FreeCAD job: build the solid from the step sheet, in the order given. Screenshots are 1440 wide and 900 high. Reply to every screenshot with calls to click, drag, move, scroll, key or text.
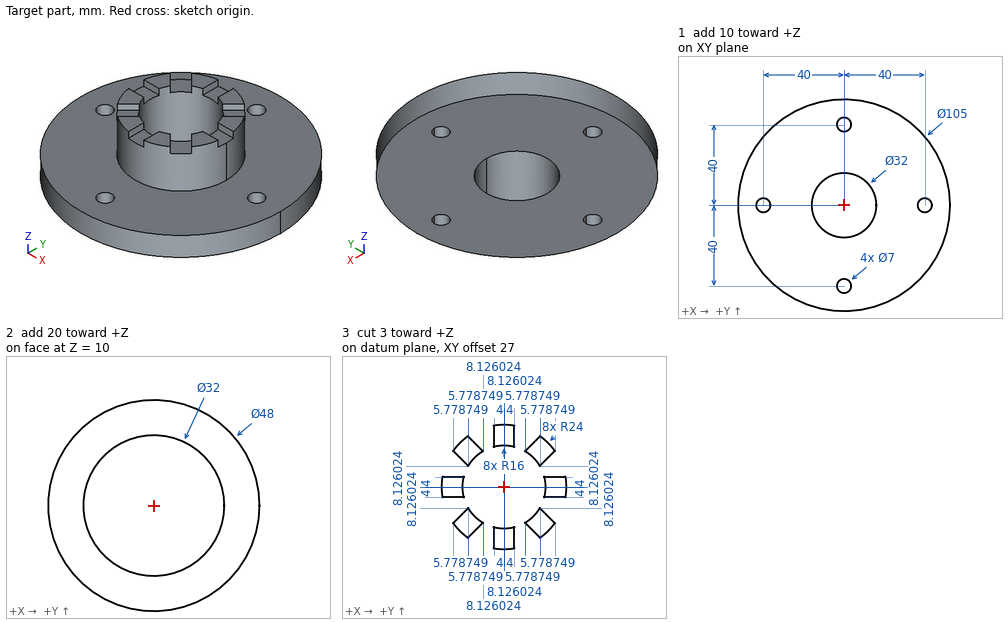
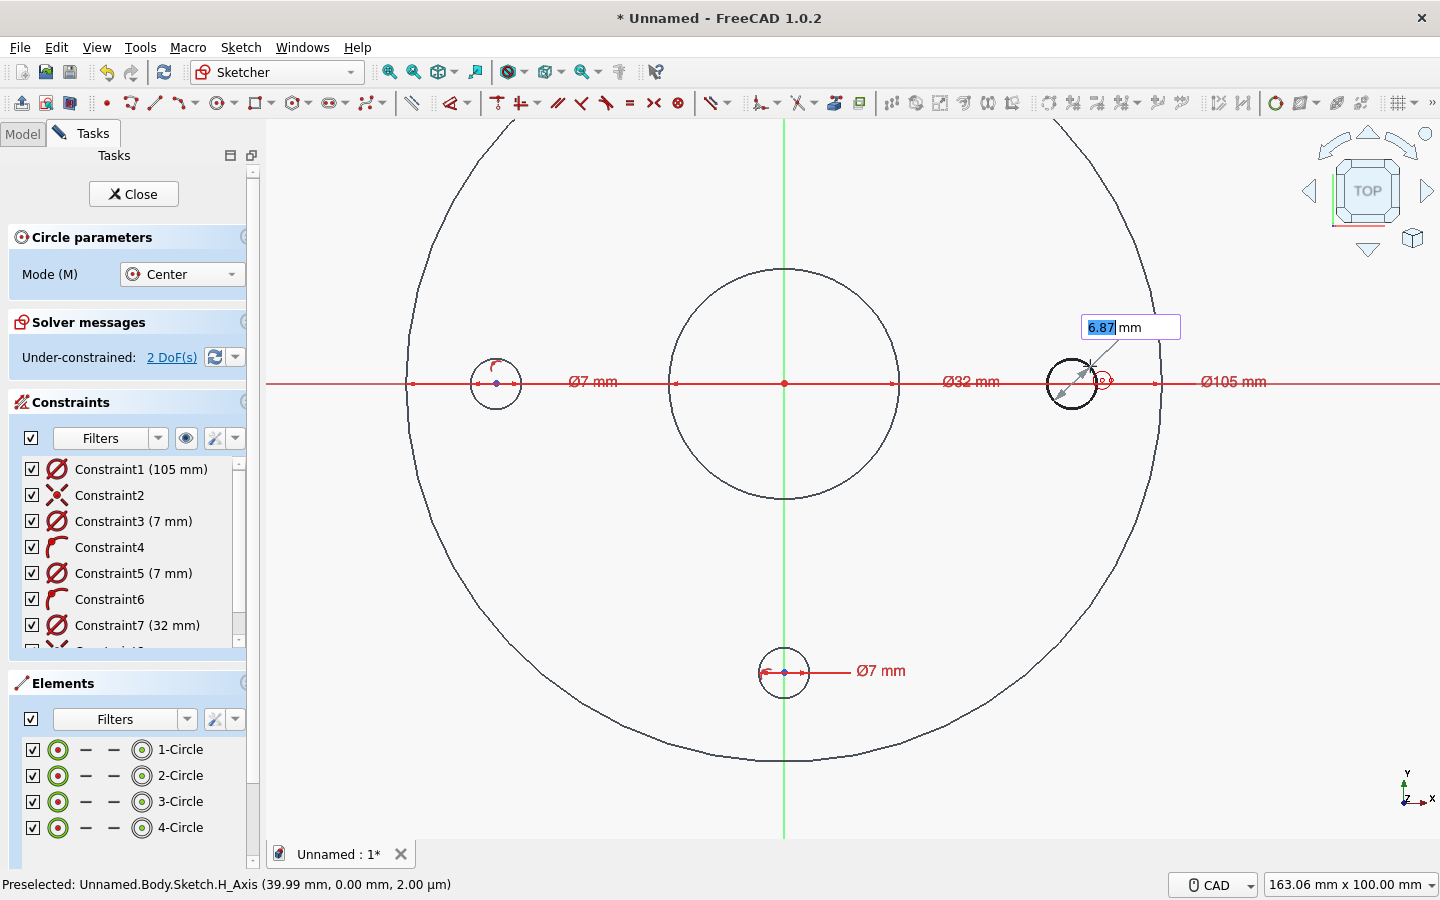
text(7)
key(Return)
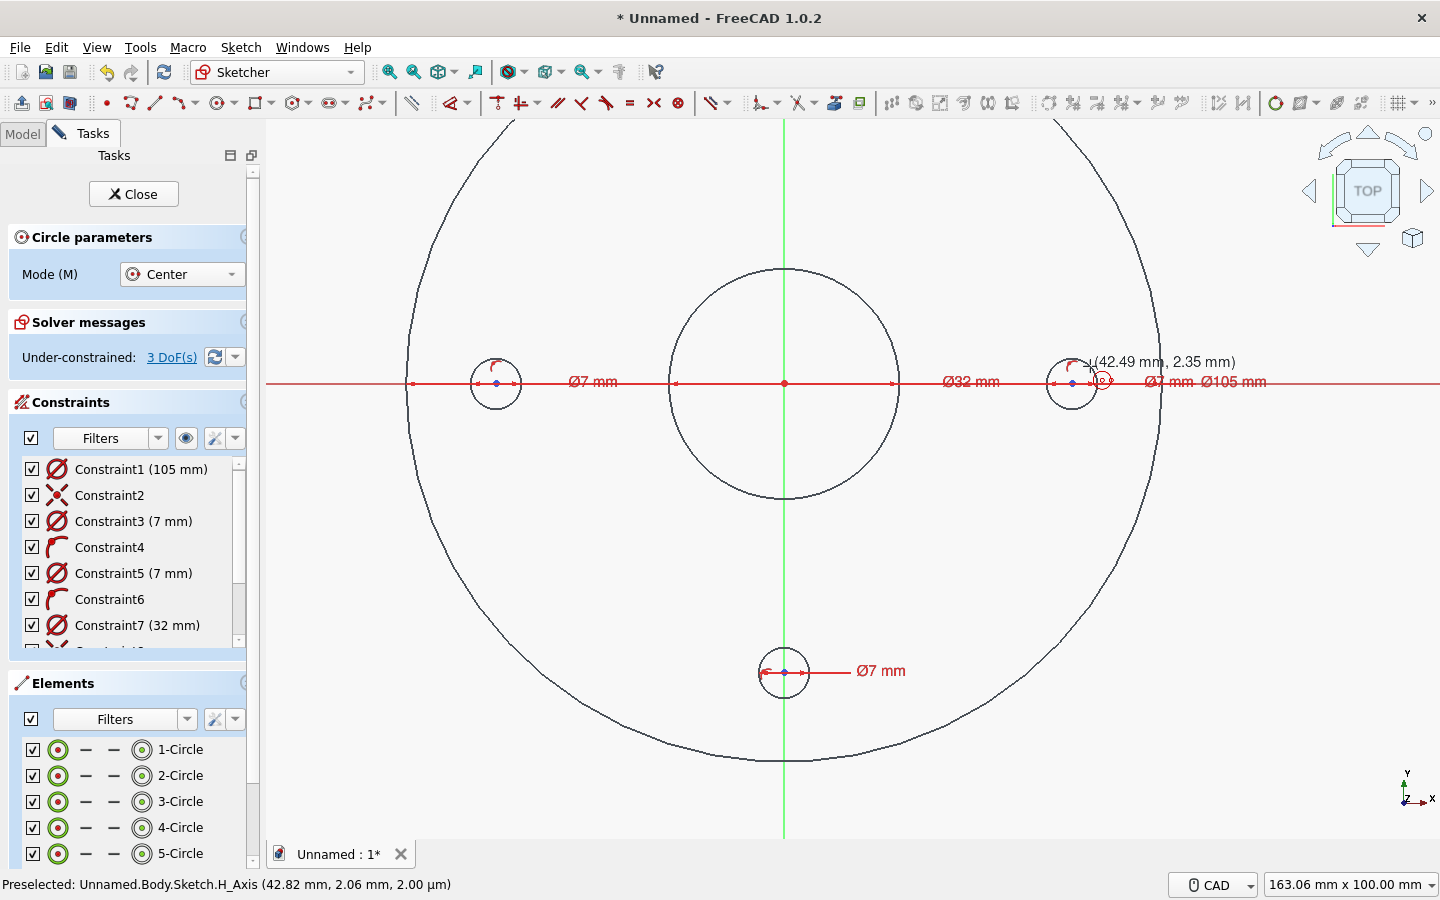
scroll(785, 672, down, 2)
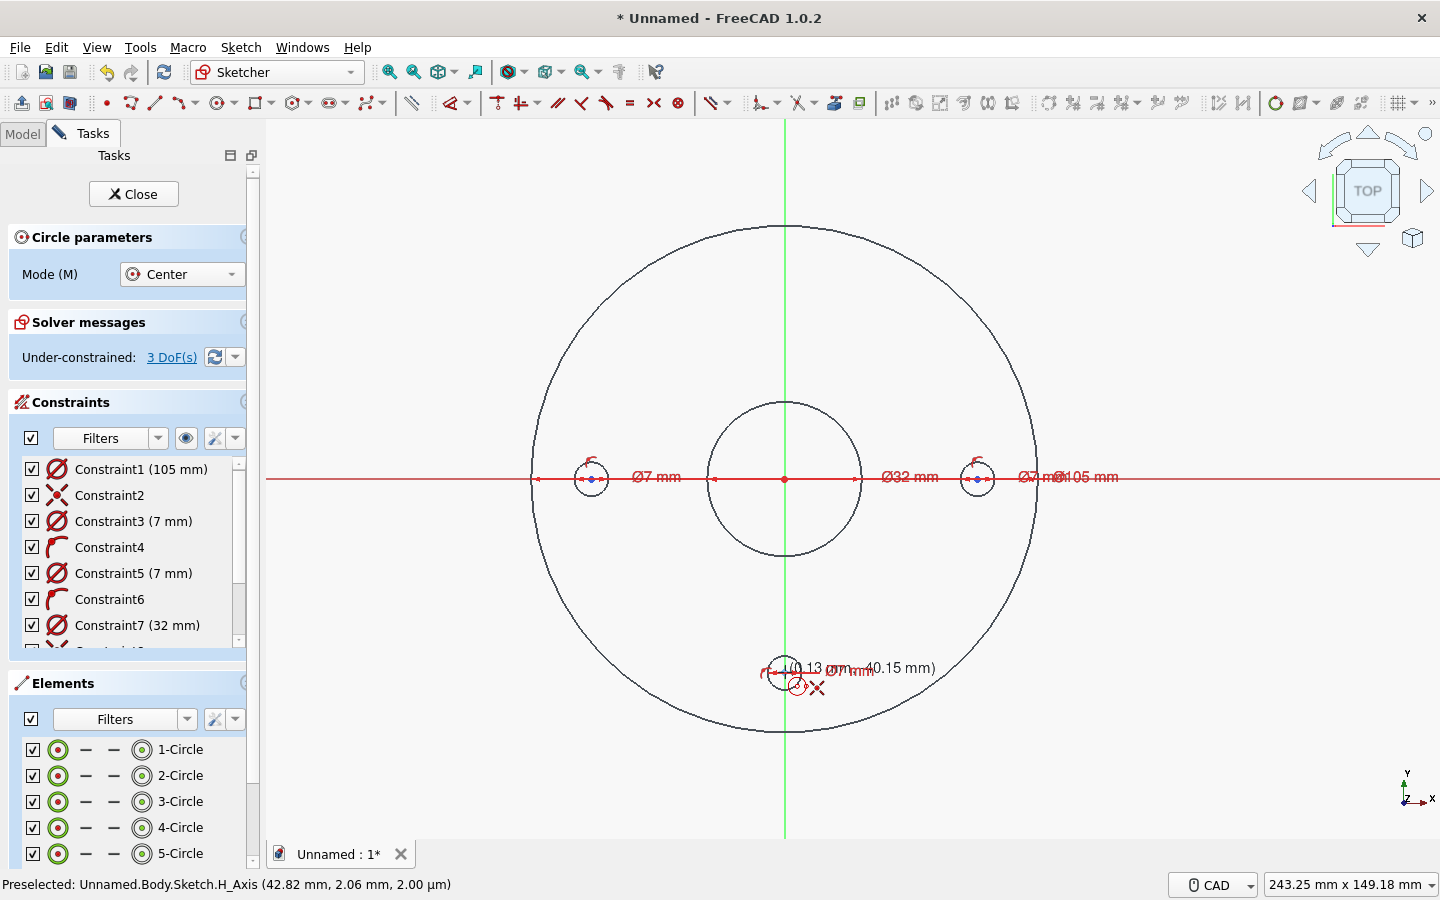
scroll(785, 286, up, 2)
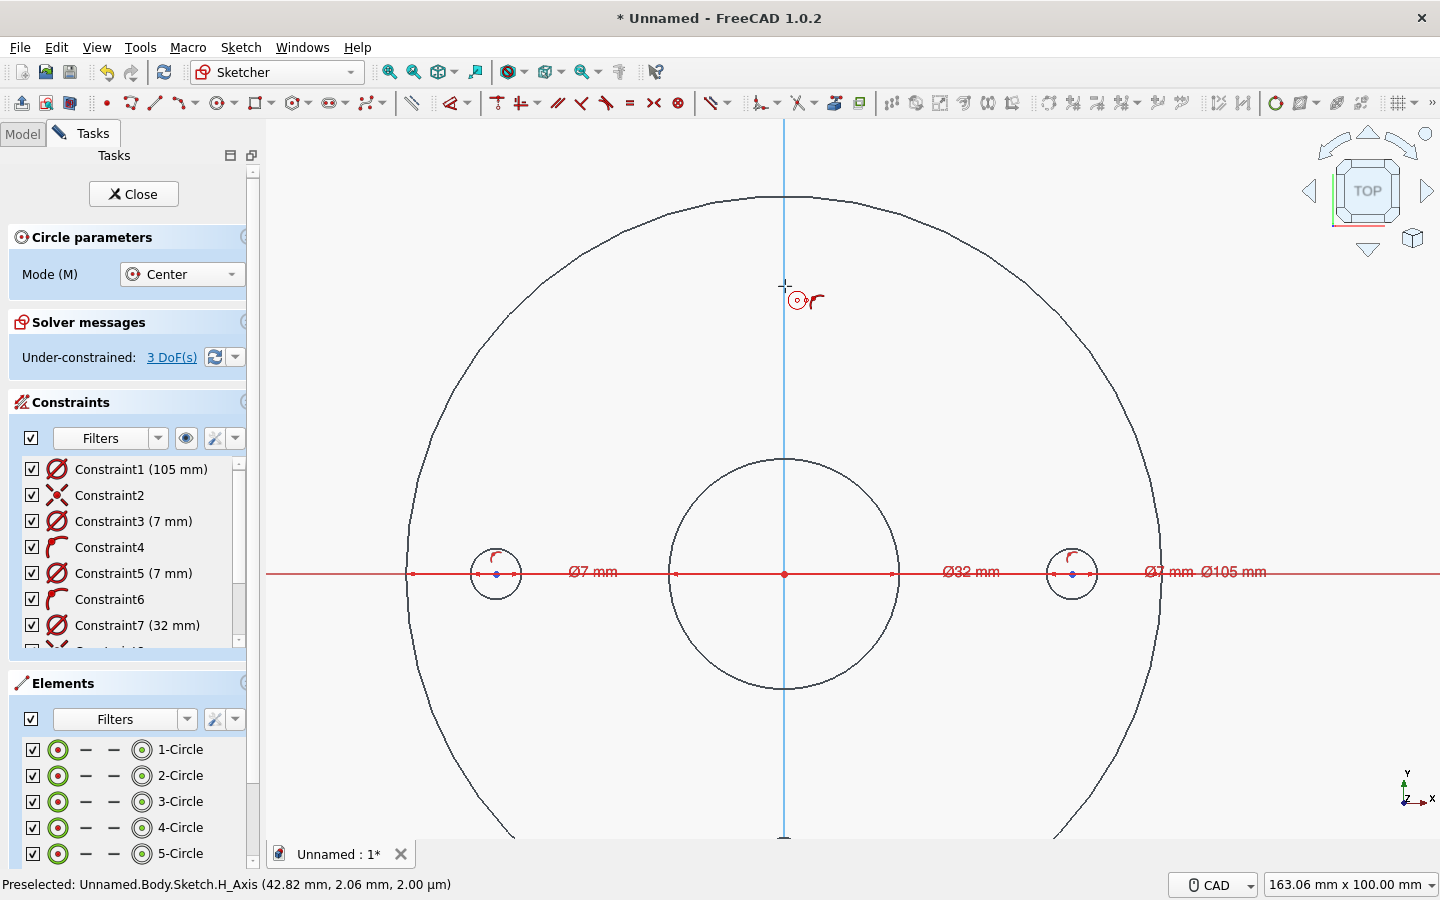
click(784, 286)
move(802, 268)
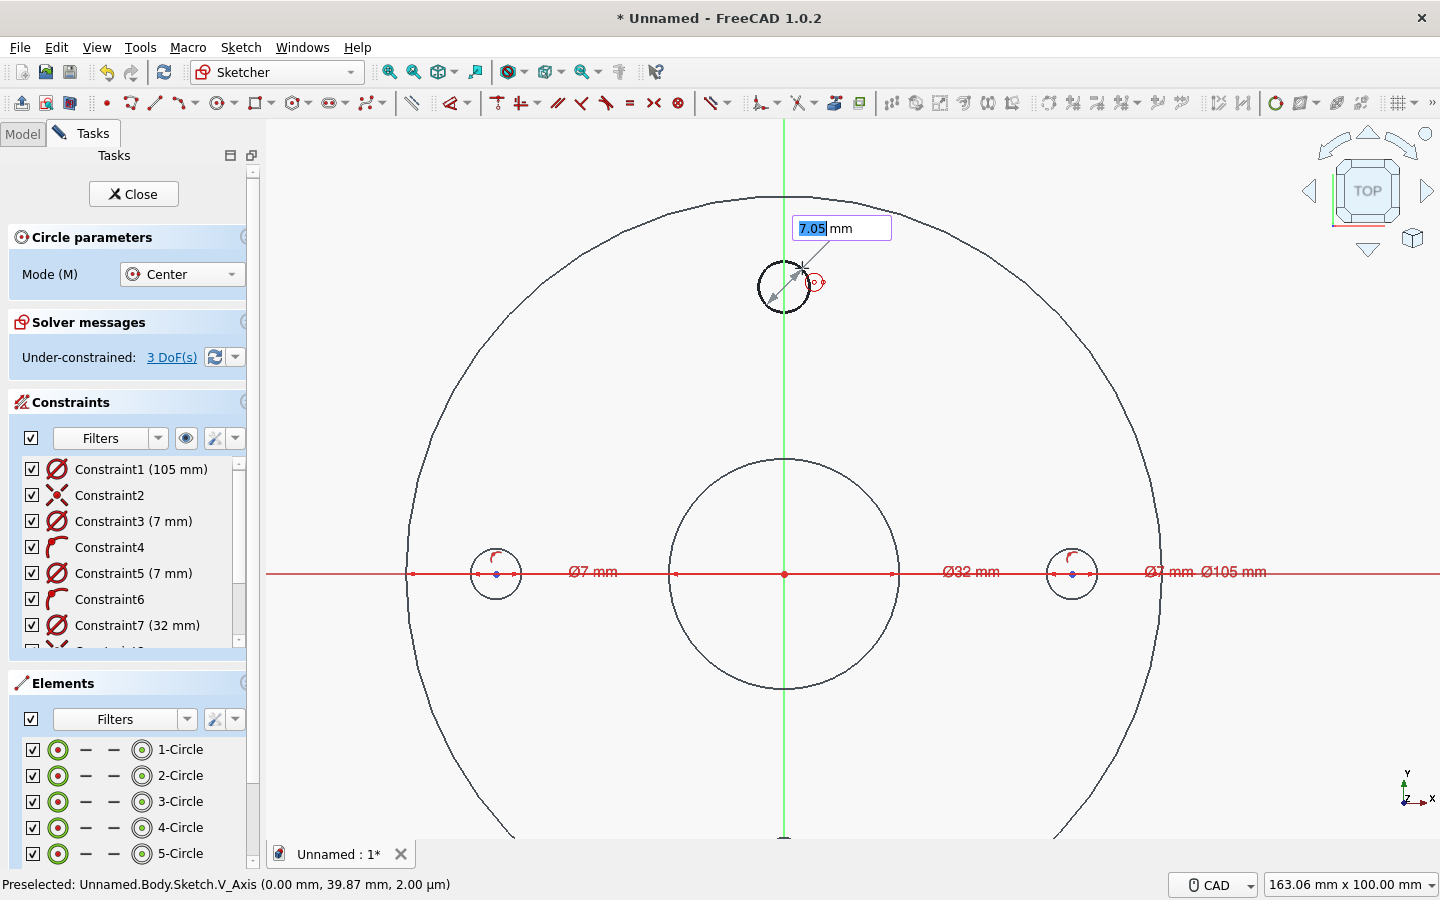
text(7)
key(Return)
key(Escape)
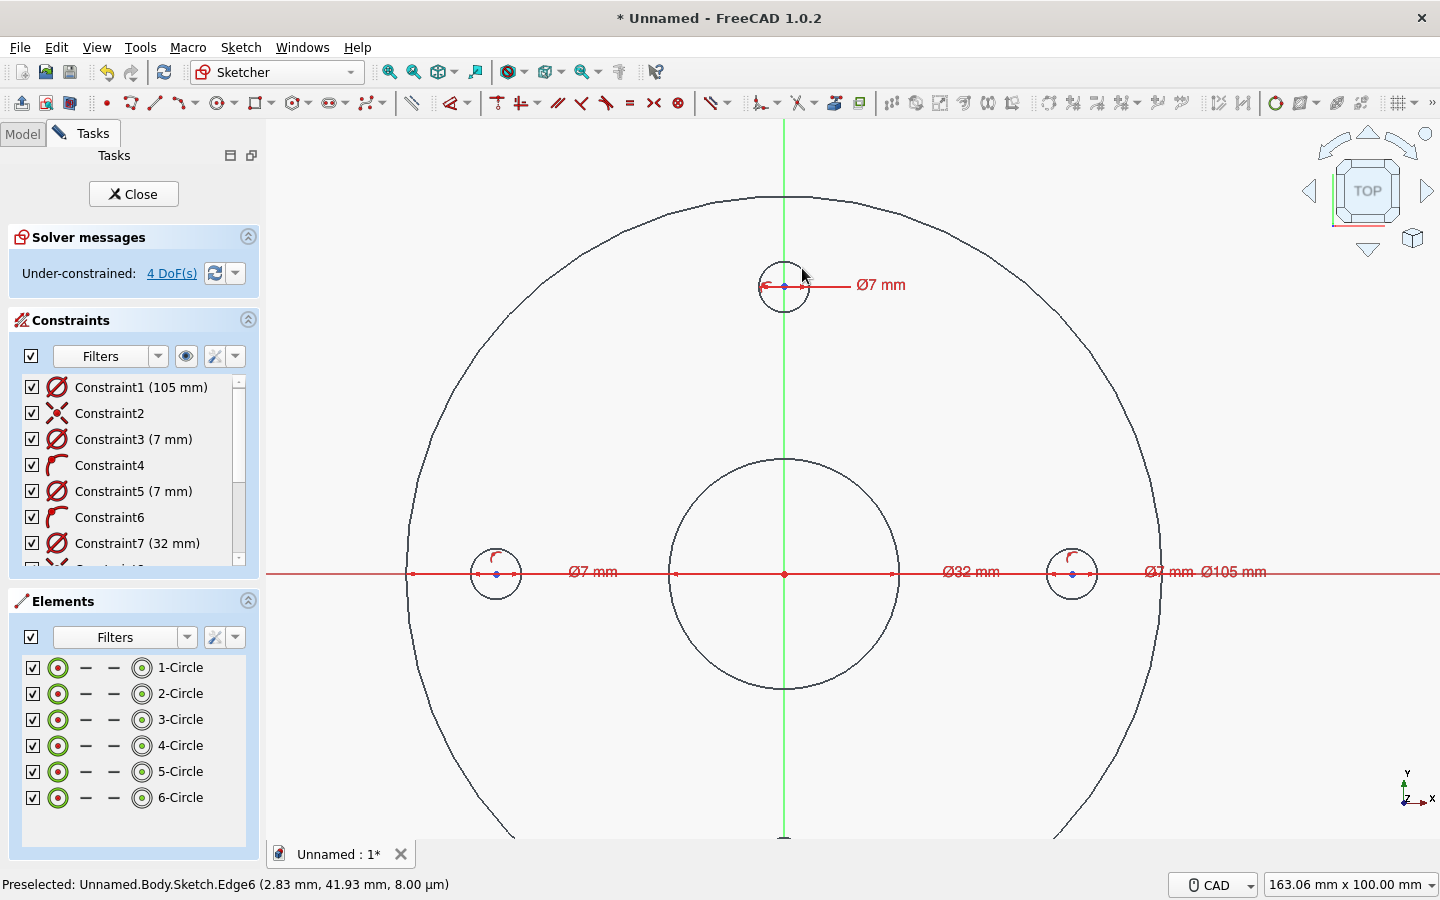
click(450, 104)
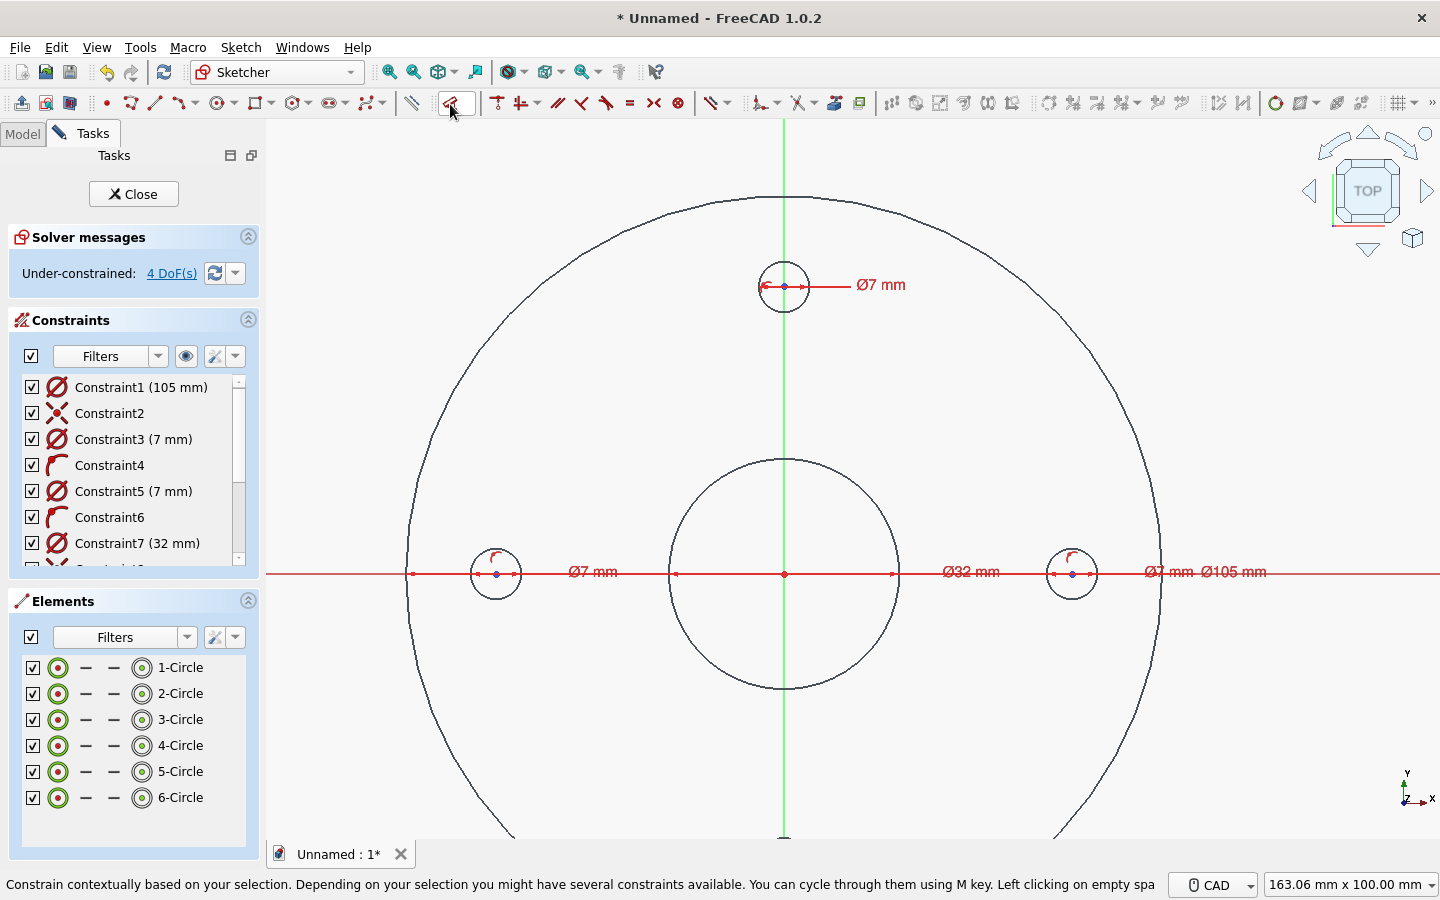
scroll(785, 286, down, 2)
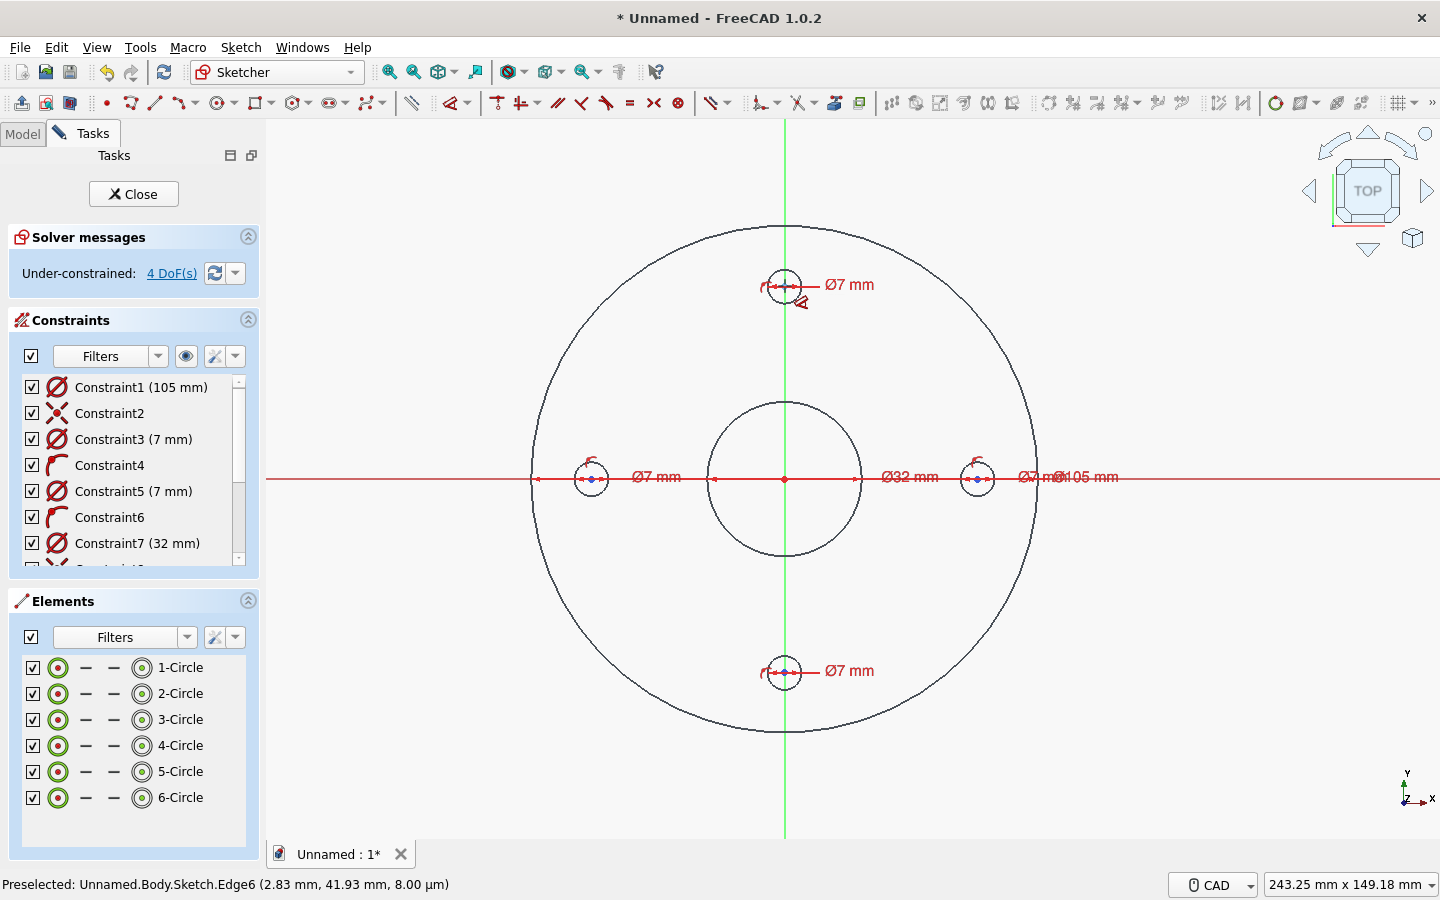
click(785, 673)
click(819, 576)